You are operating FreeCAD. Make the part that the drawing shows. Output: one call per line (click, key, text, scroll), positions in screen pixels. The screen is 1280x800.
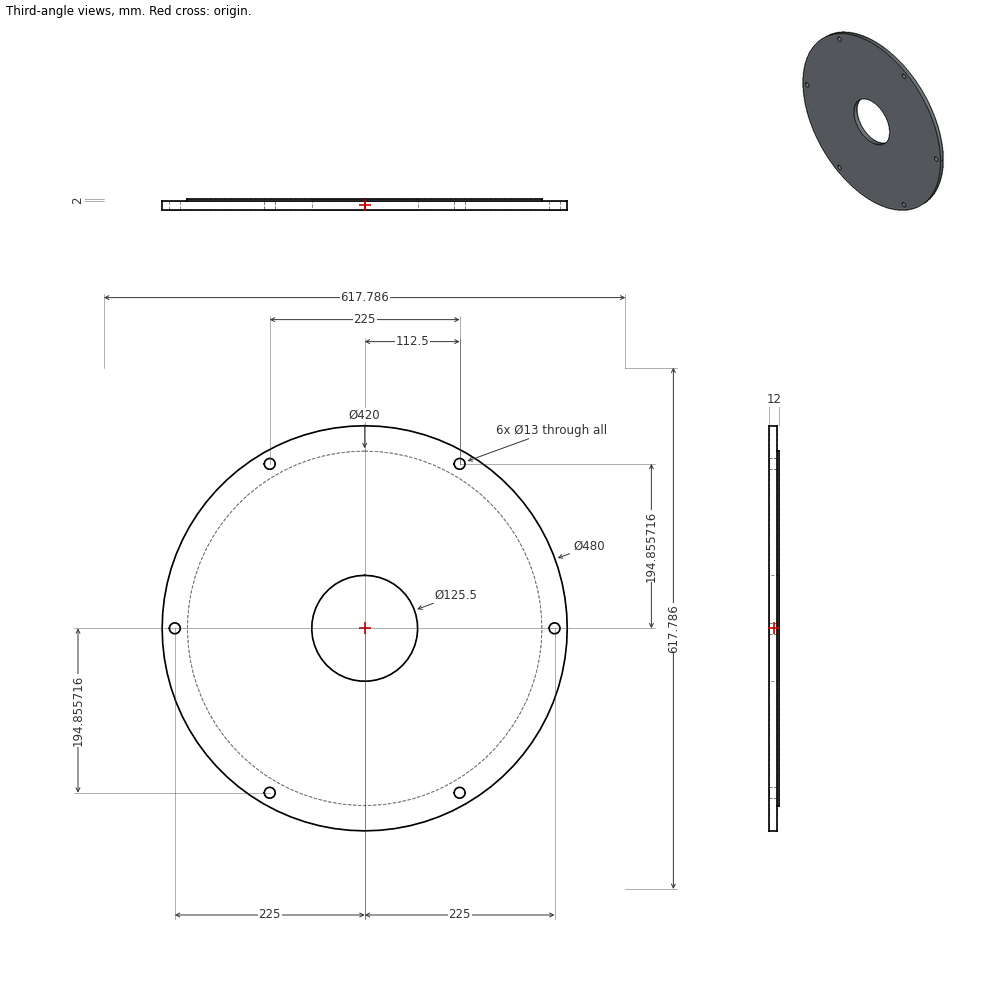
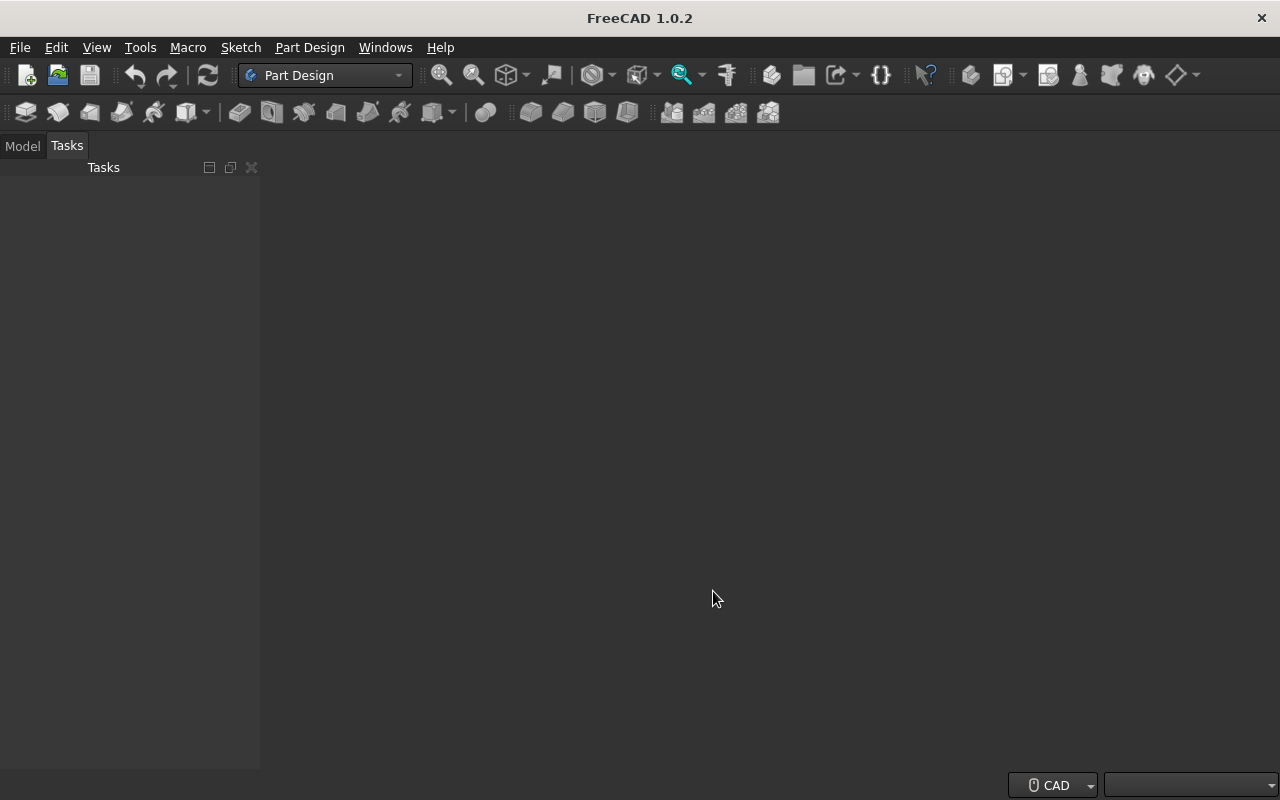
click(26, 76)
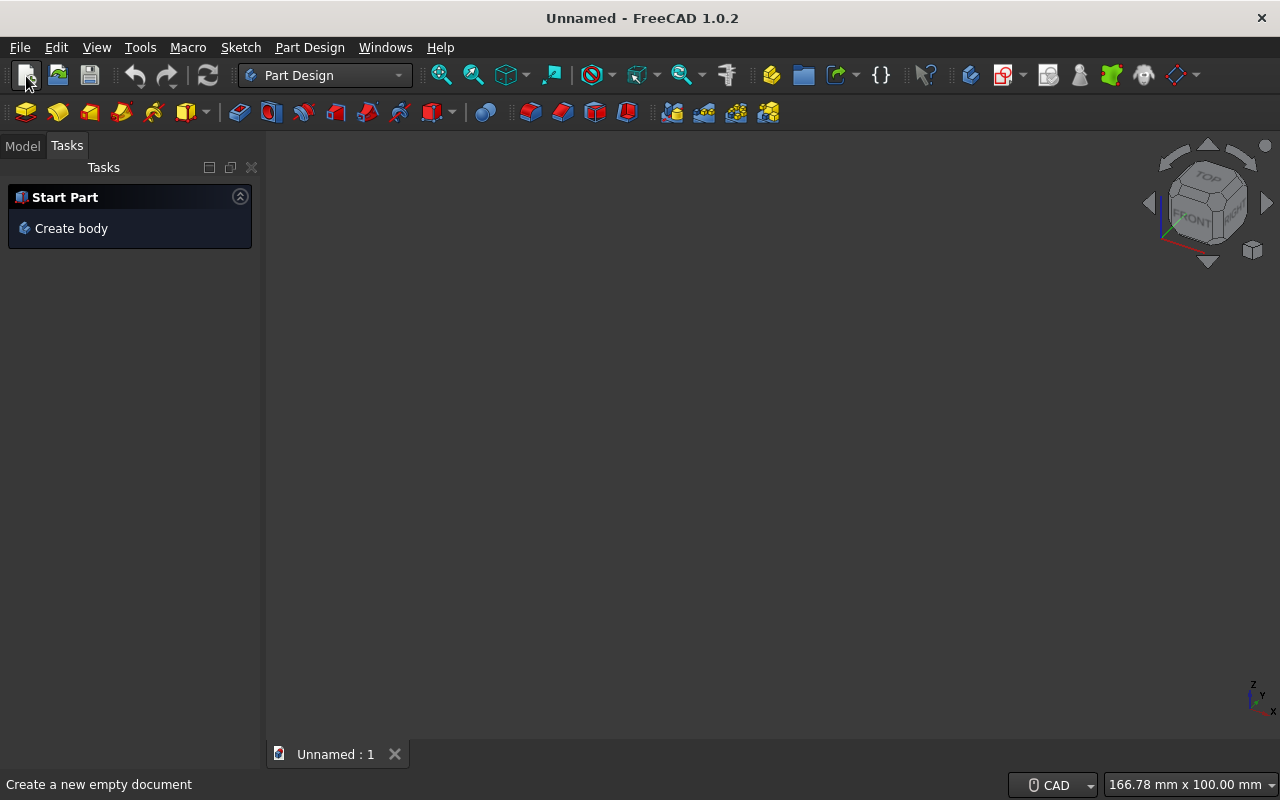
click(1004, 76)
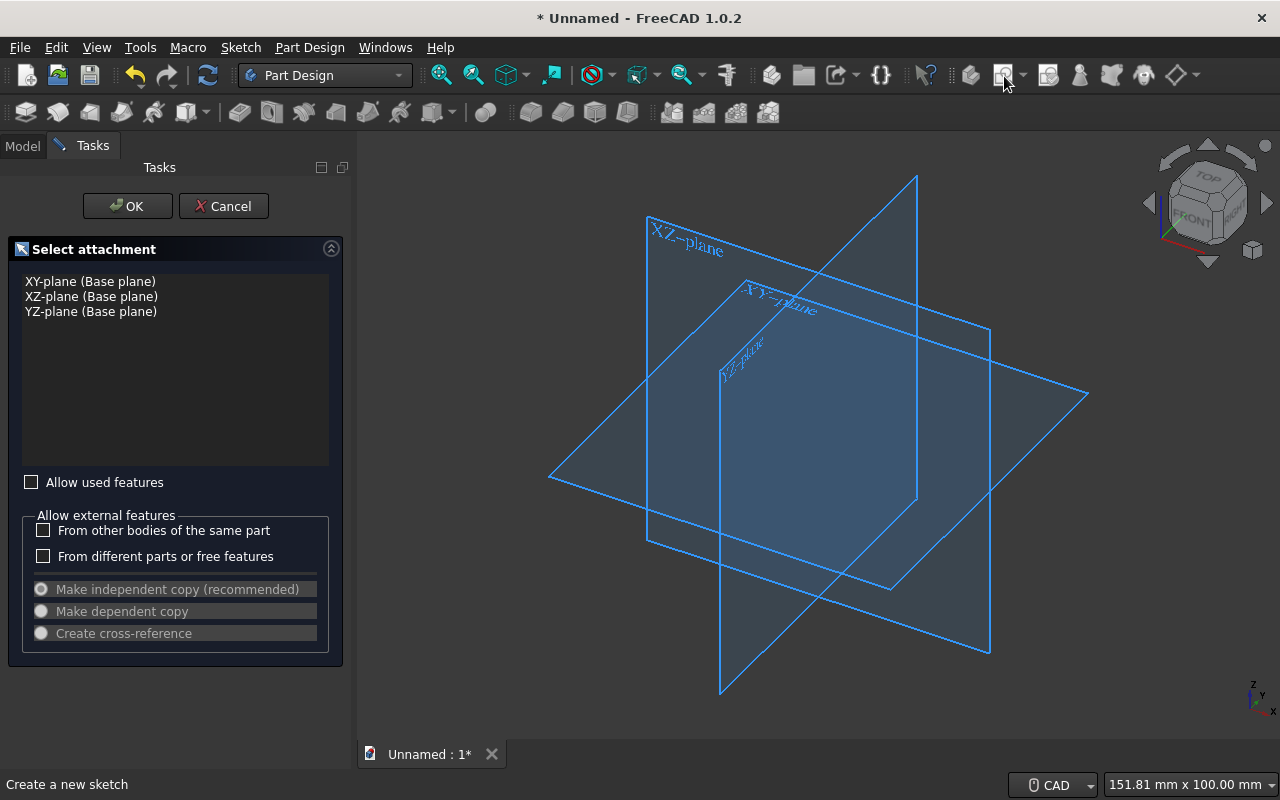
click(82, 296)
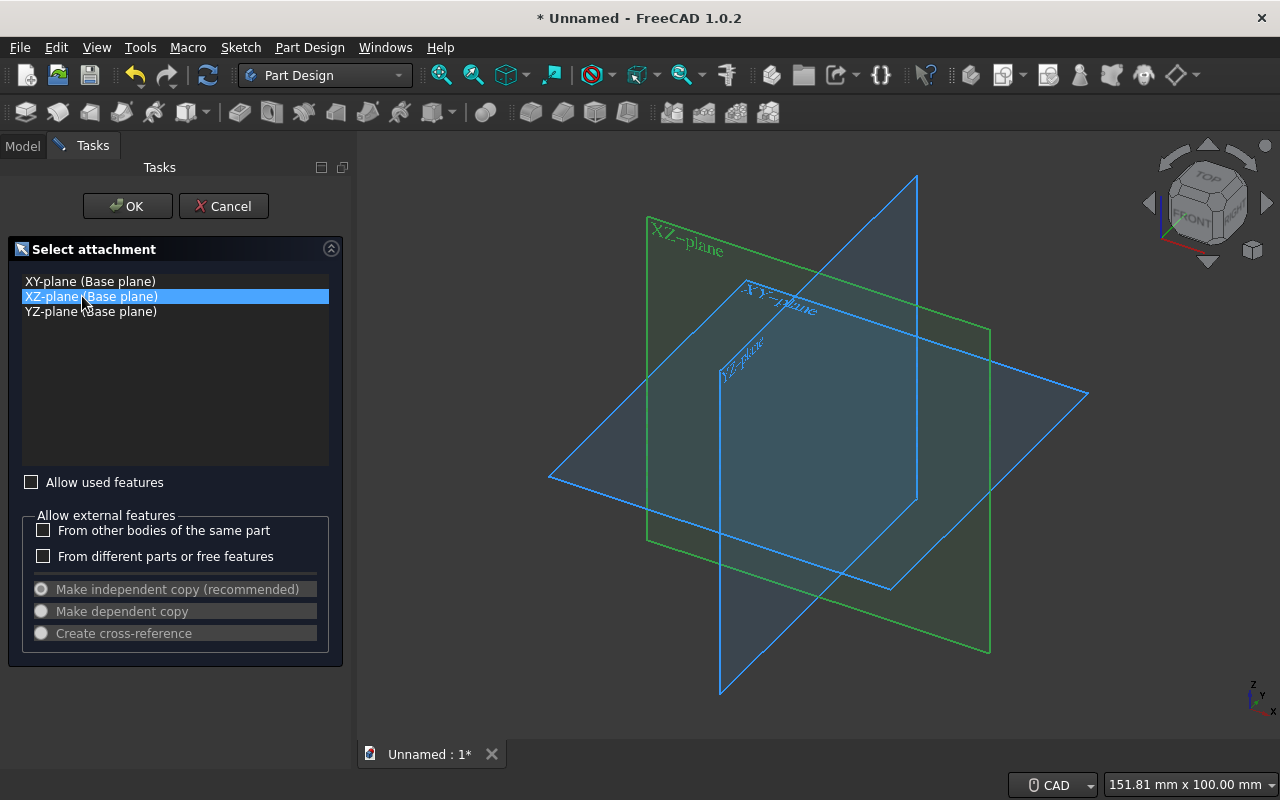
click(128, 206)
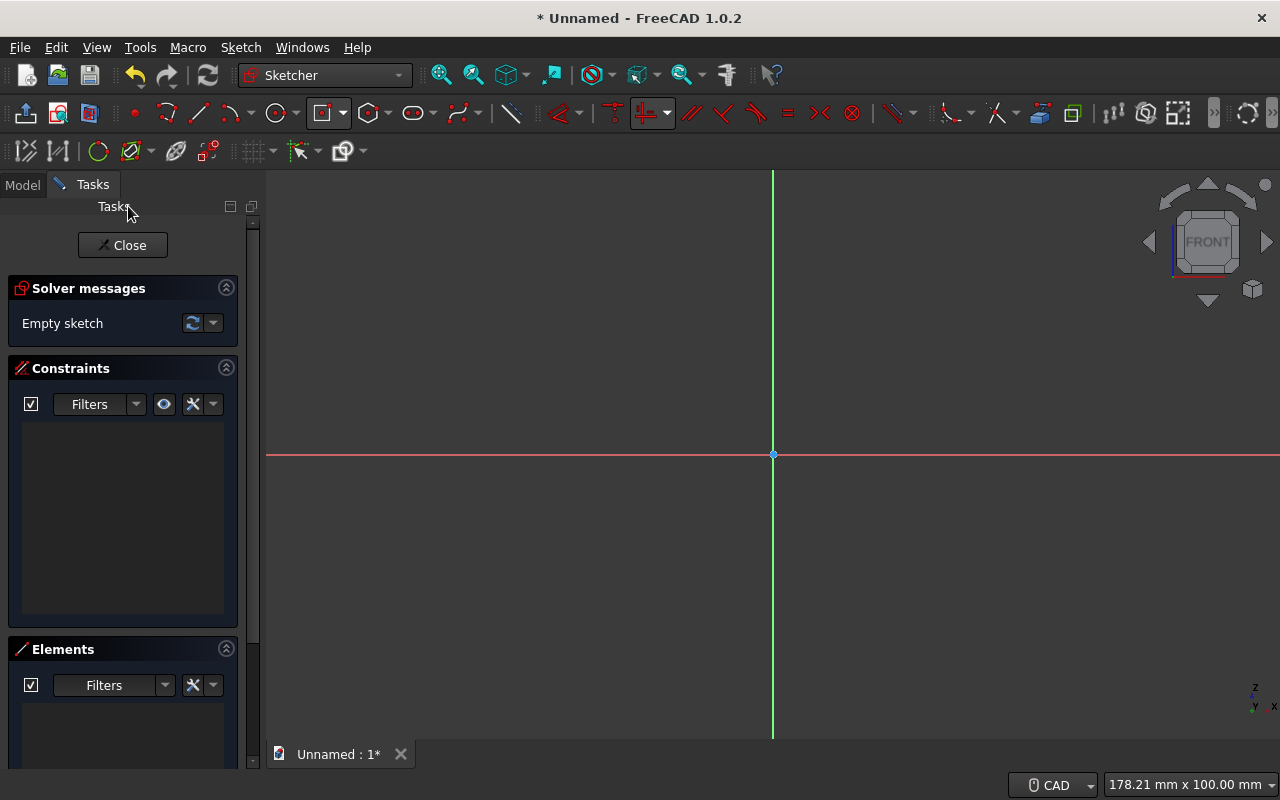
scroll(694, 454, down, 10)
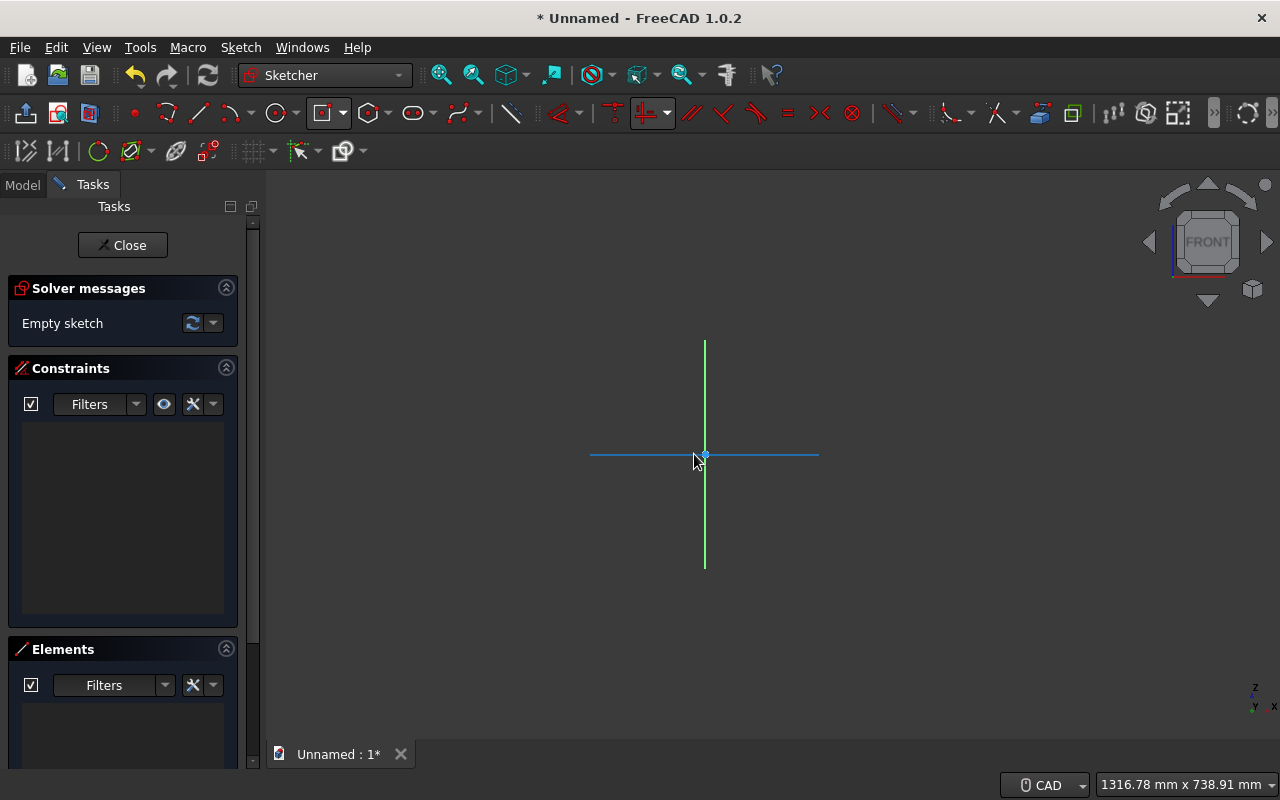
click(276, 114)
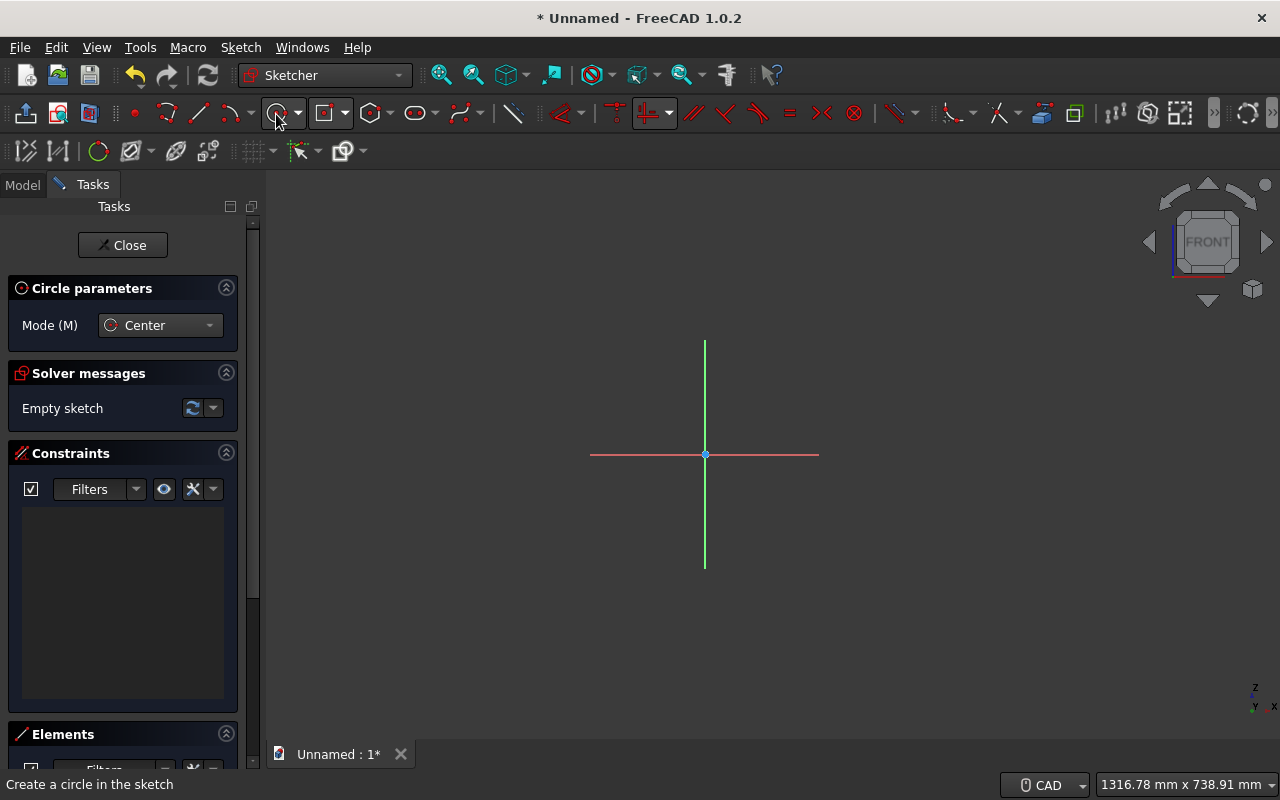
click(705, 454)
move(836, 324)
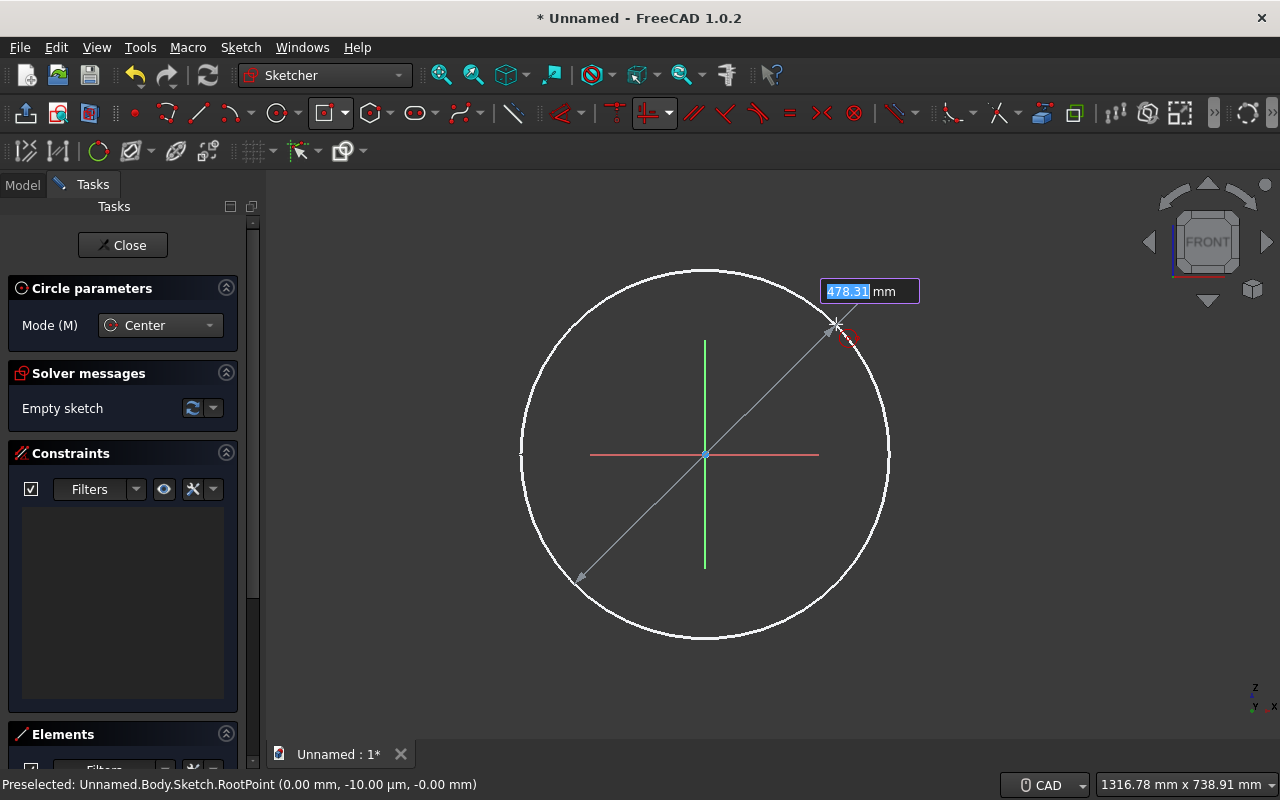
text(480)
key(Return)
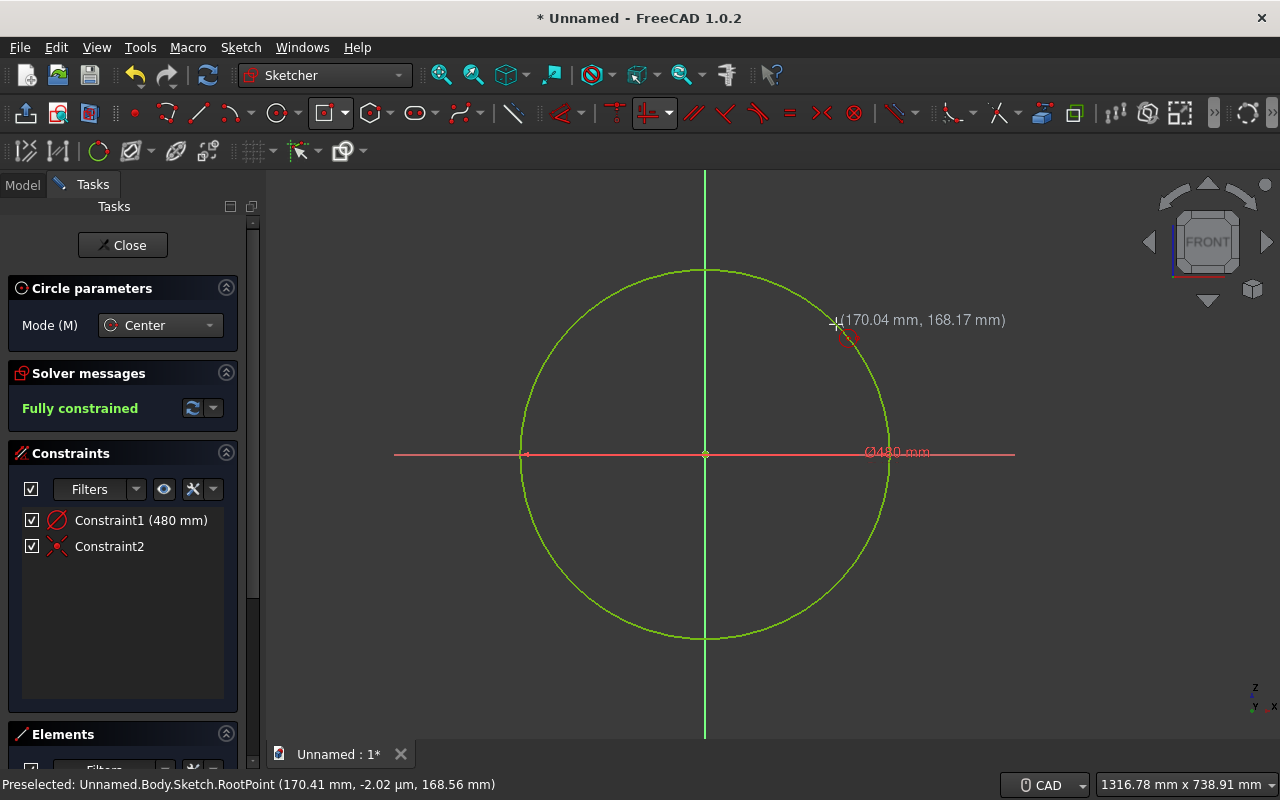
click(705, 454)
move(739, 420)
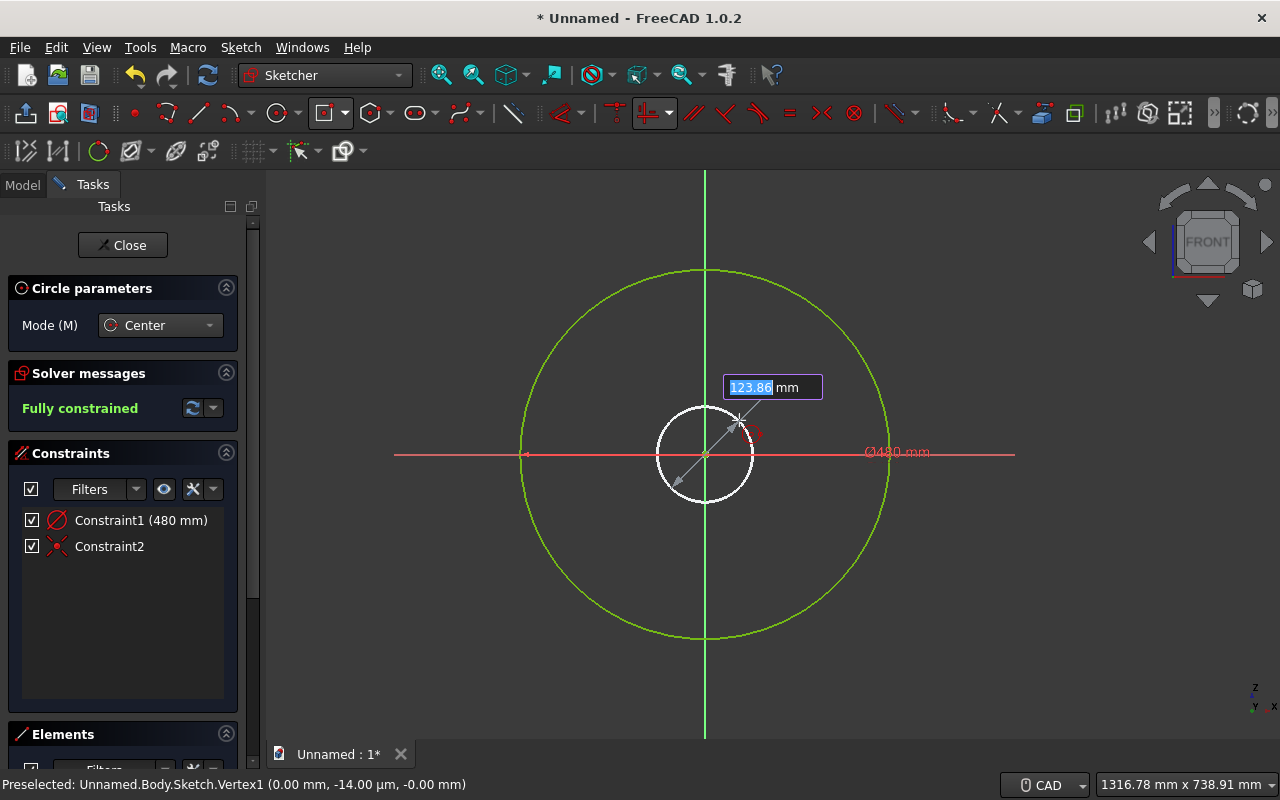
text(125.5)
key(Return)
key(Escape)